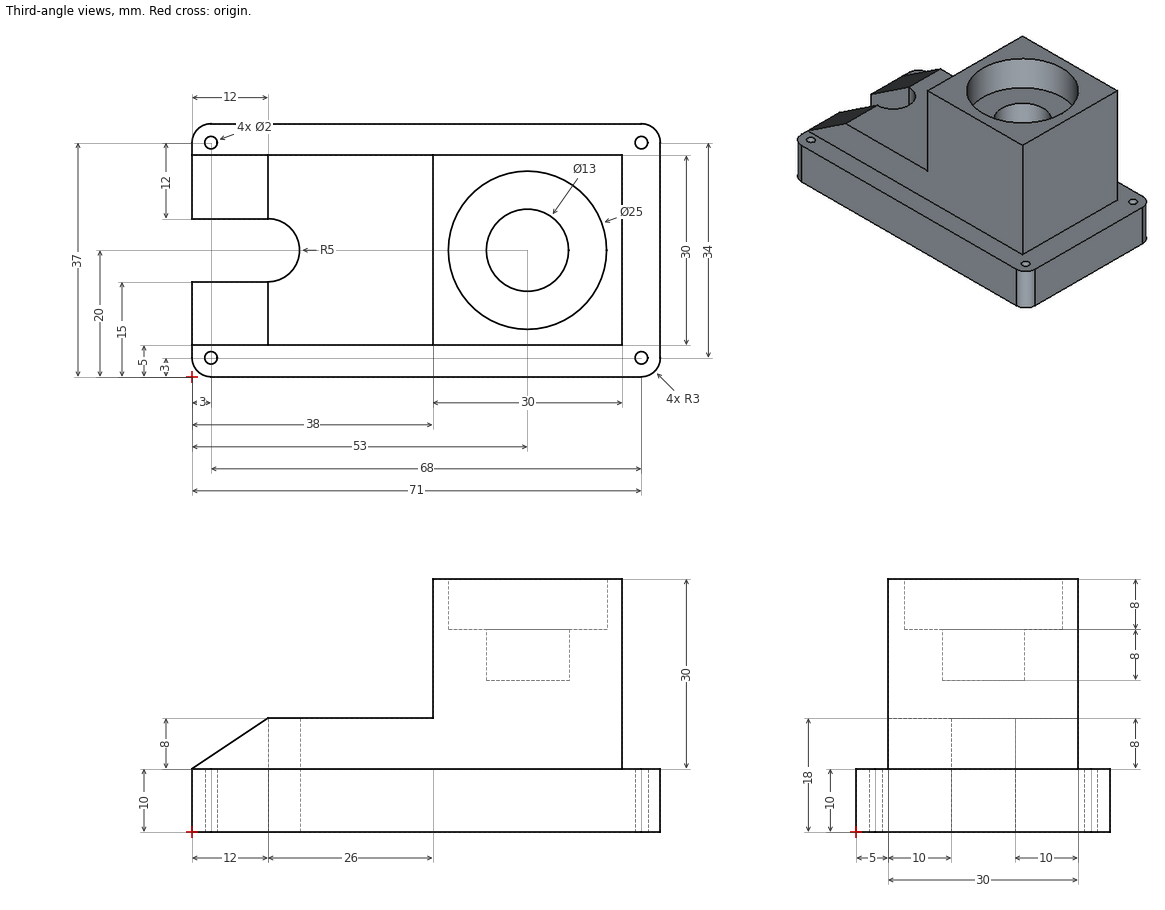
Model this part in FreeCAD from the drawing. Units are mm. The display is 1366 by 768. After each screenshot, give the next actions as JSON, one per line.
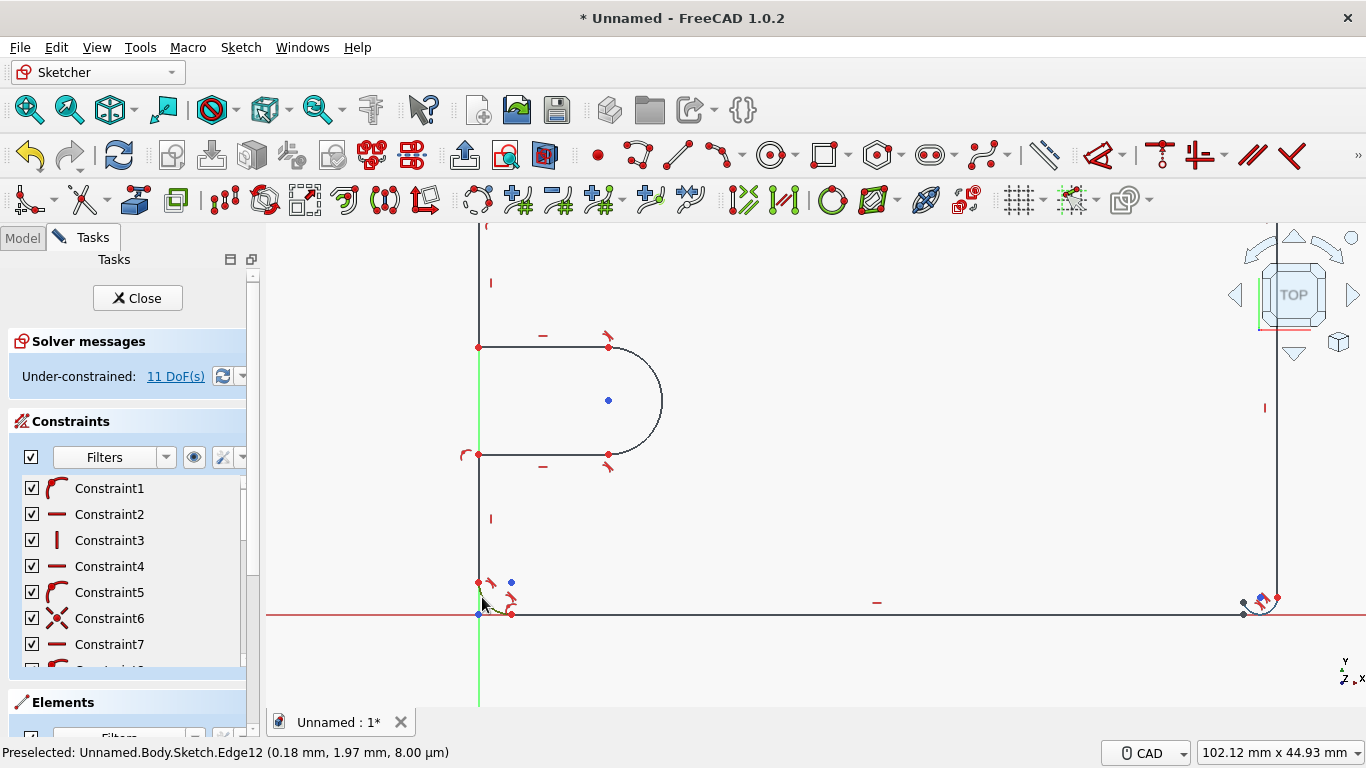
{"action": "key", "text": "e"}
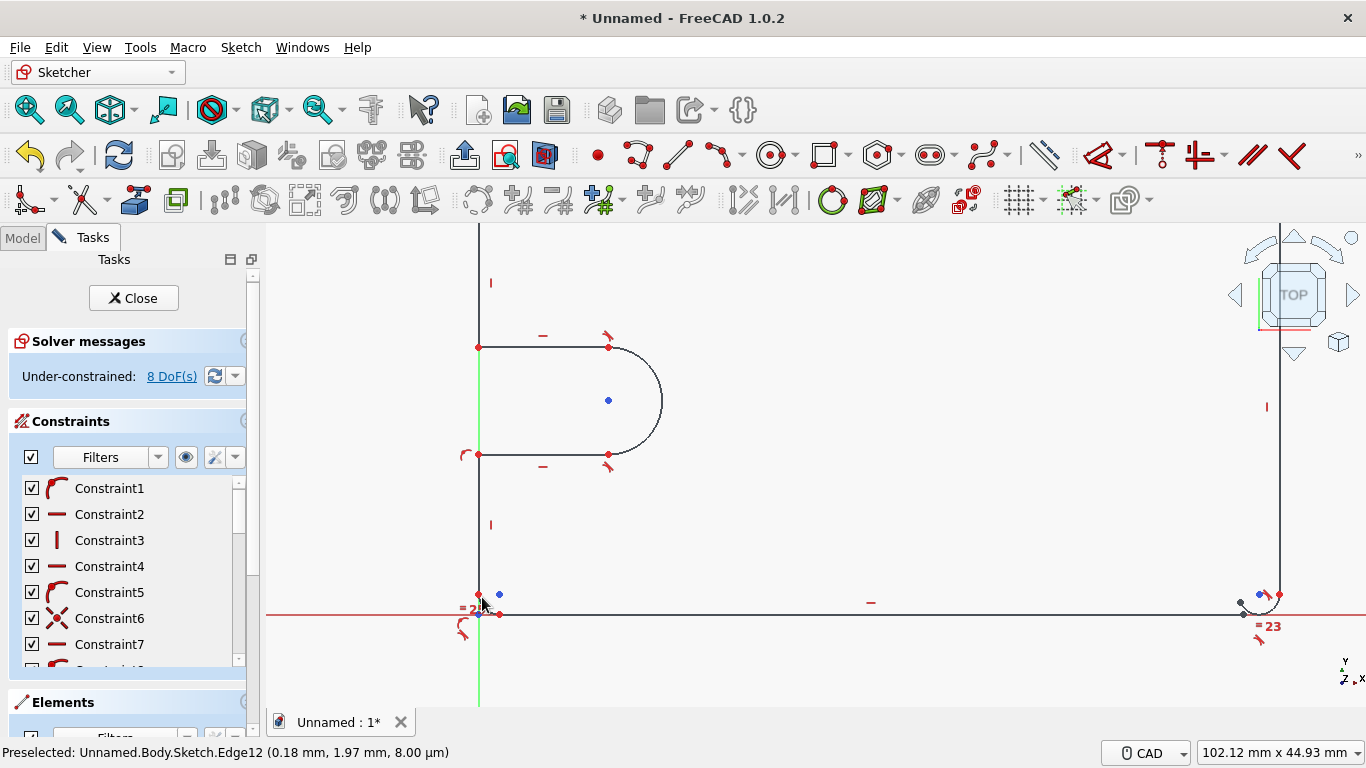
{"action": "left_click", "coordinate": [1098, 156]}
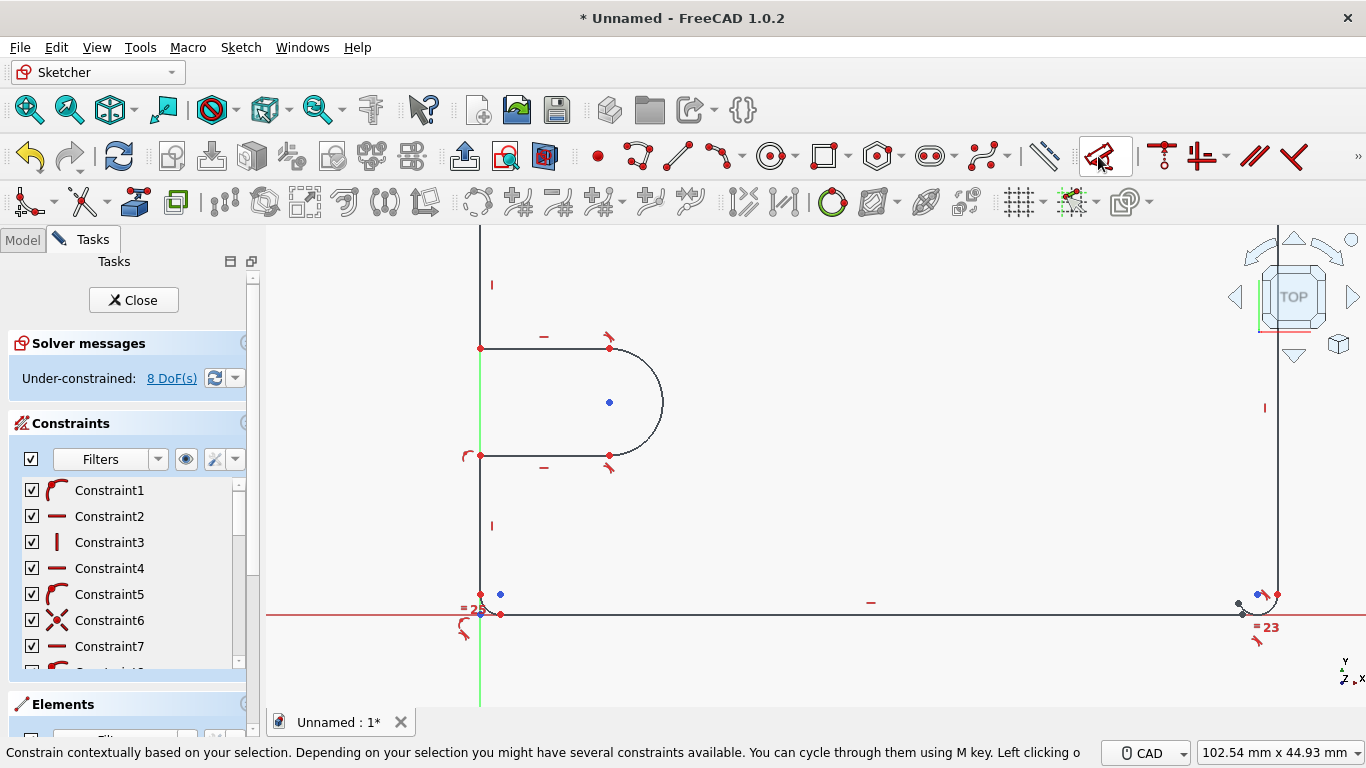
{"action": "scroll", "coordinate": [484, 599], "scroll_direction": "down", "scroll_amount": 2}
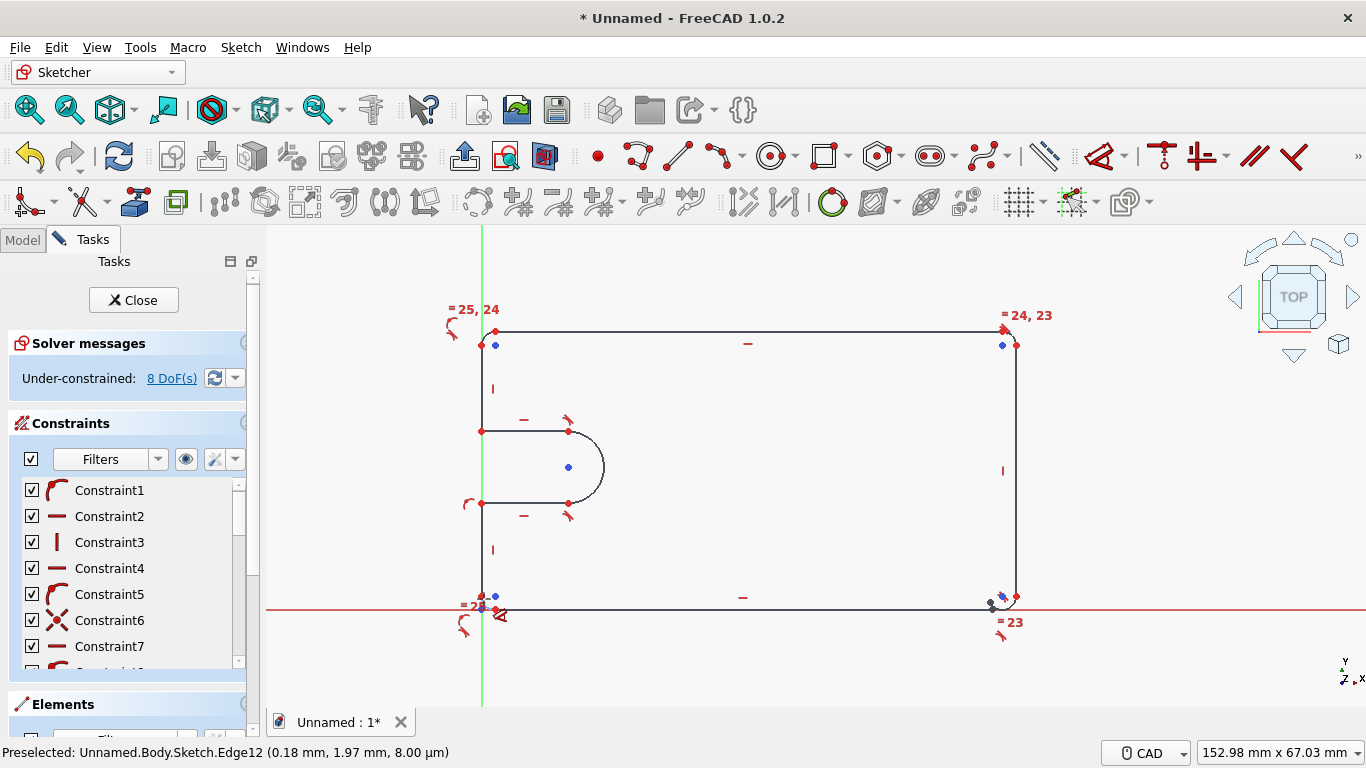
{"action": "scroll", "coordinate": [1005, 610], "scroll_direction": "up", "scroll_amount": 4}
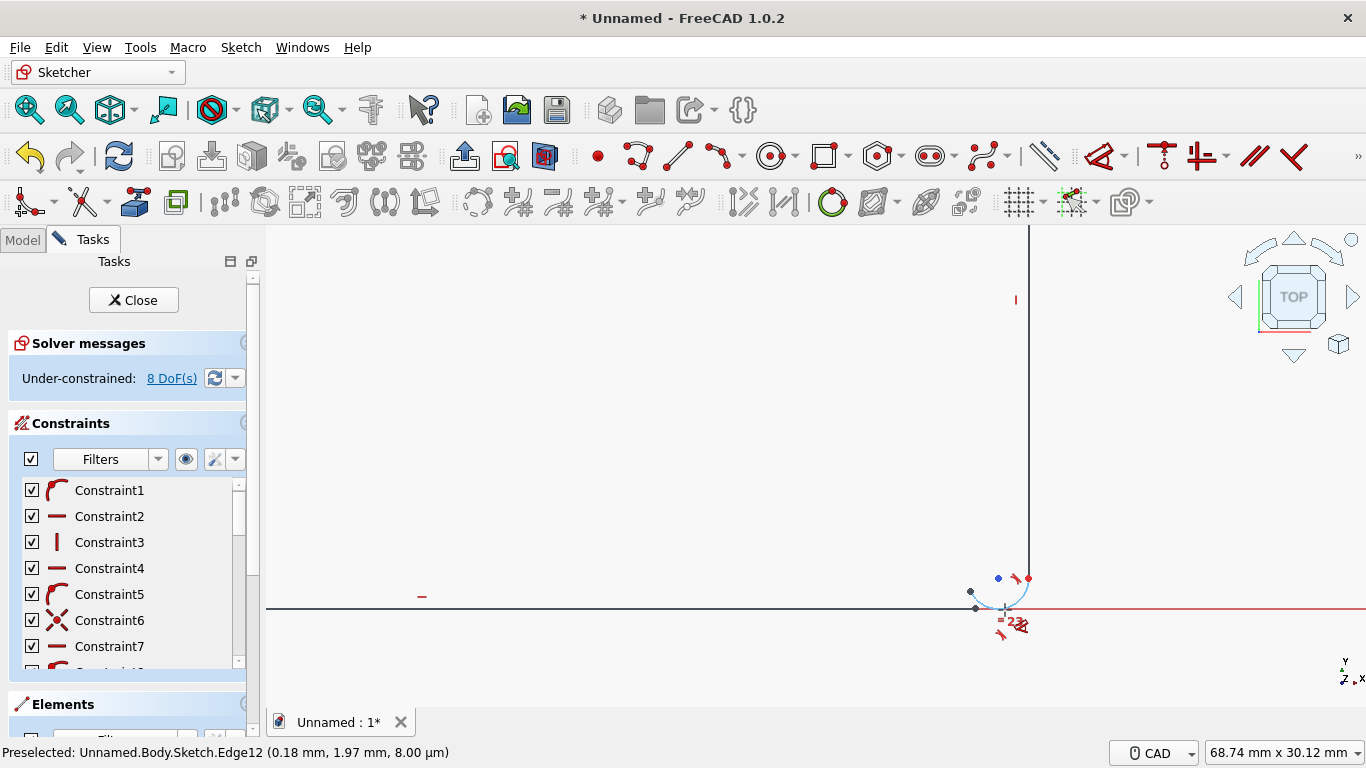
{"action": "left_click", "coordinate": [1005, 608]}
{"action": "left_click", "coordinate": [1012, 639]}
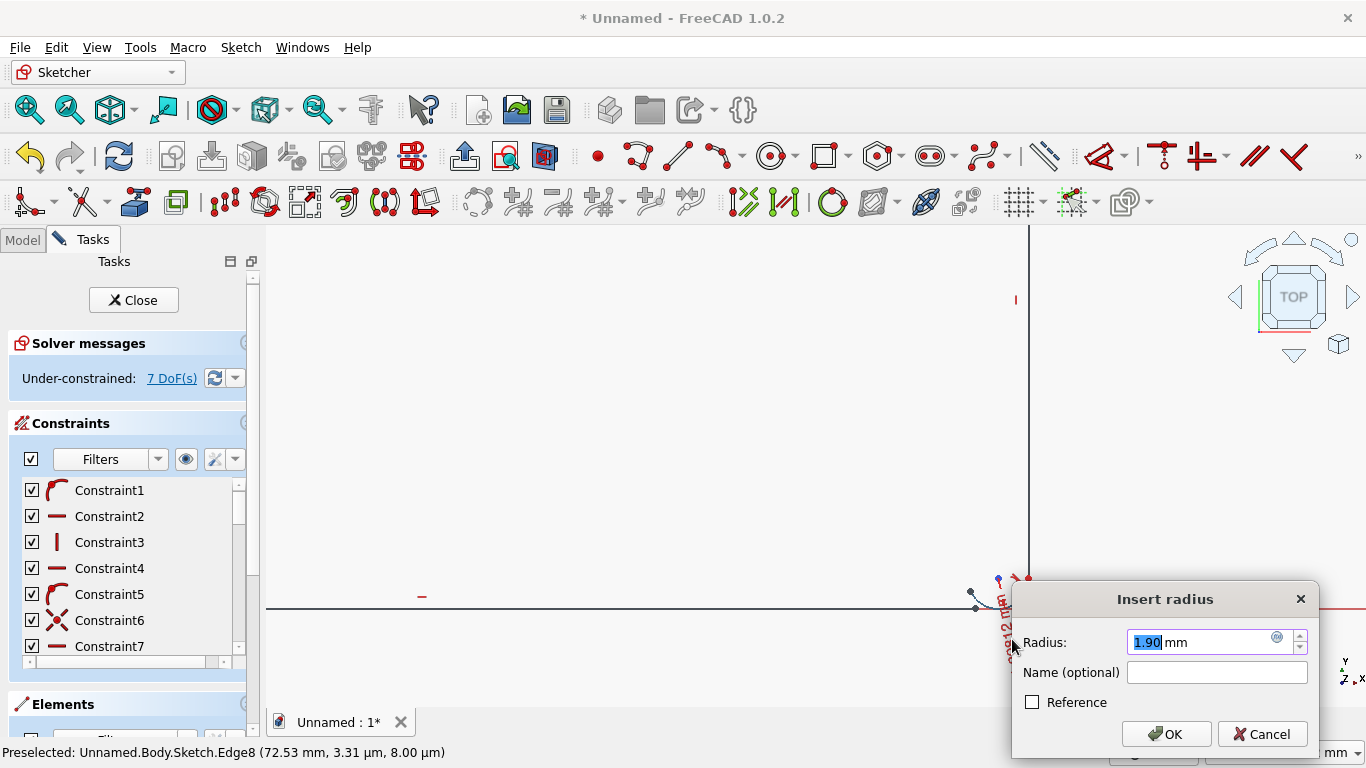
{"action": "type", "text": "3"}
{"action": "key", "text": "Return"}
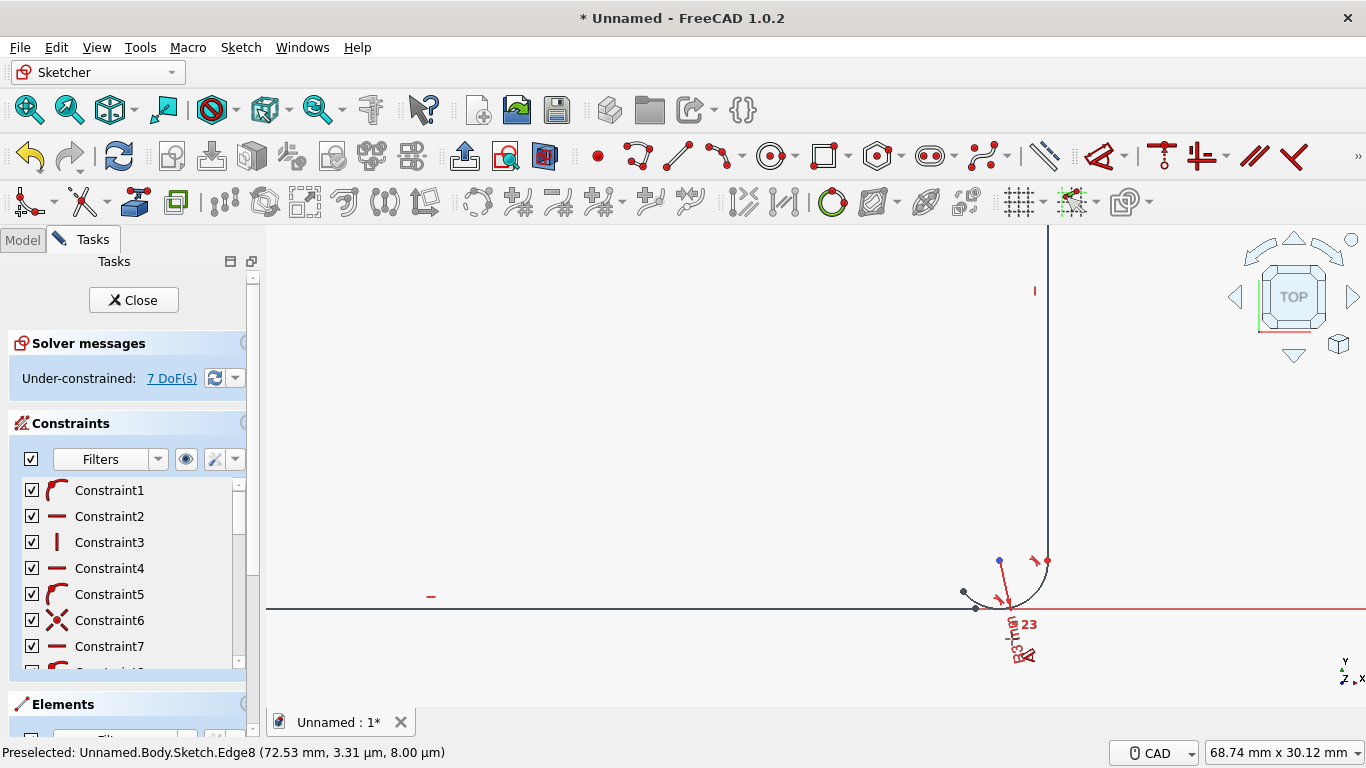
{"action": "scroll", "coordinate": [1005, 611], "scroll_direction": "down", "scroll_amount": 4}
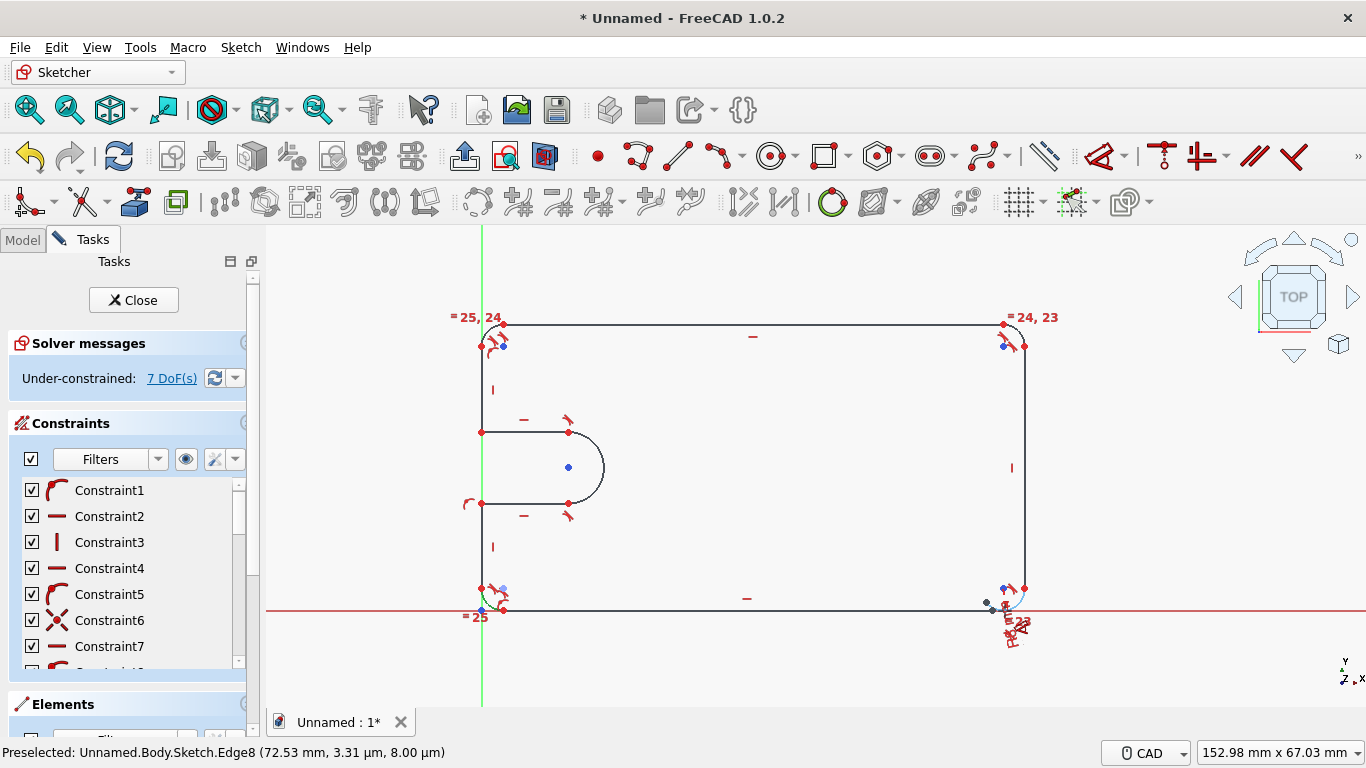
{"action": "left_click", "coordinate": [597, 489]}
{"action": "left_click", "coordinate": [623, 508]}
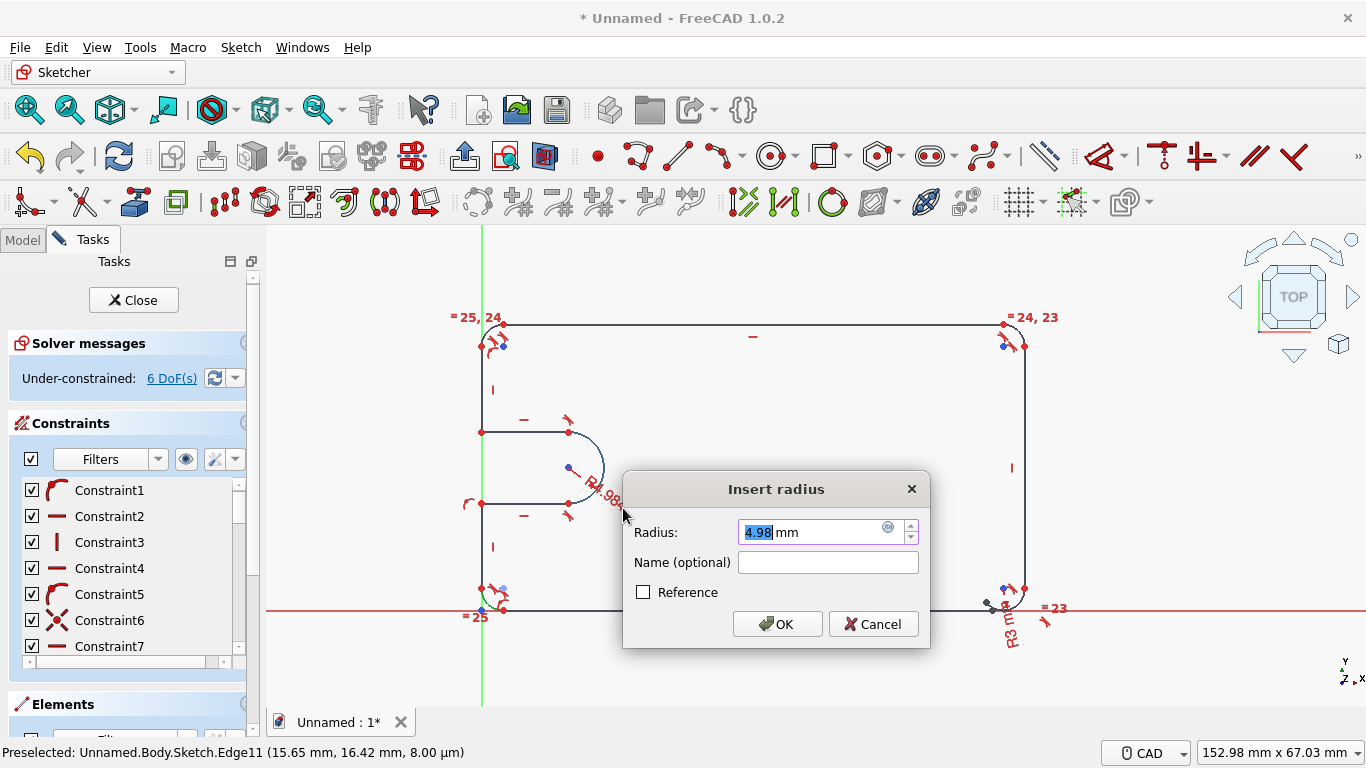
{"action": "type", "text": "5"}
{"action": "key", "text": "Return"}